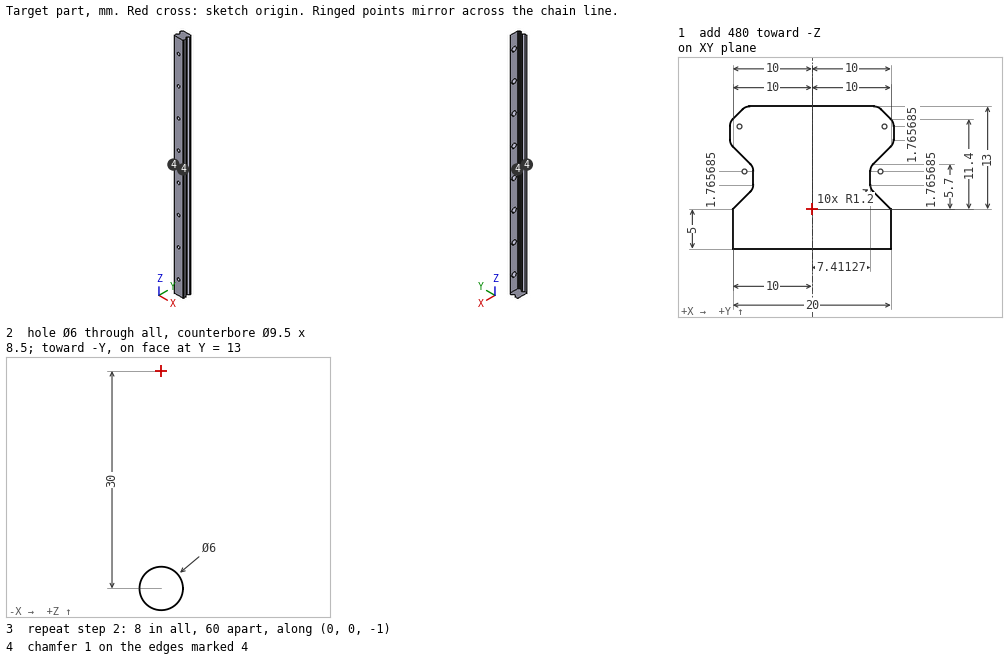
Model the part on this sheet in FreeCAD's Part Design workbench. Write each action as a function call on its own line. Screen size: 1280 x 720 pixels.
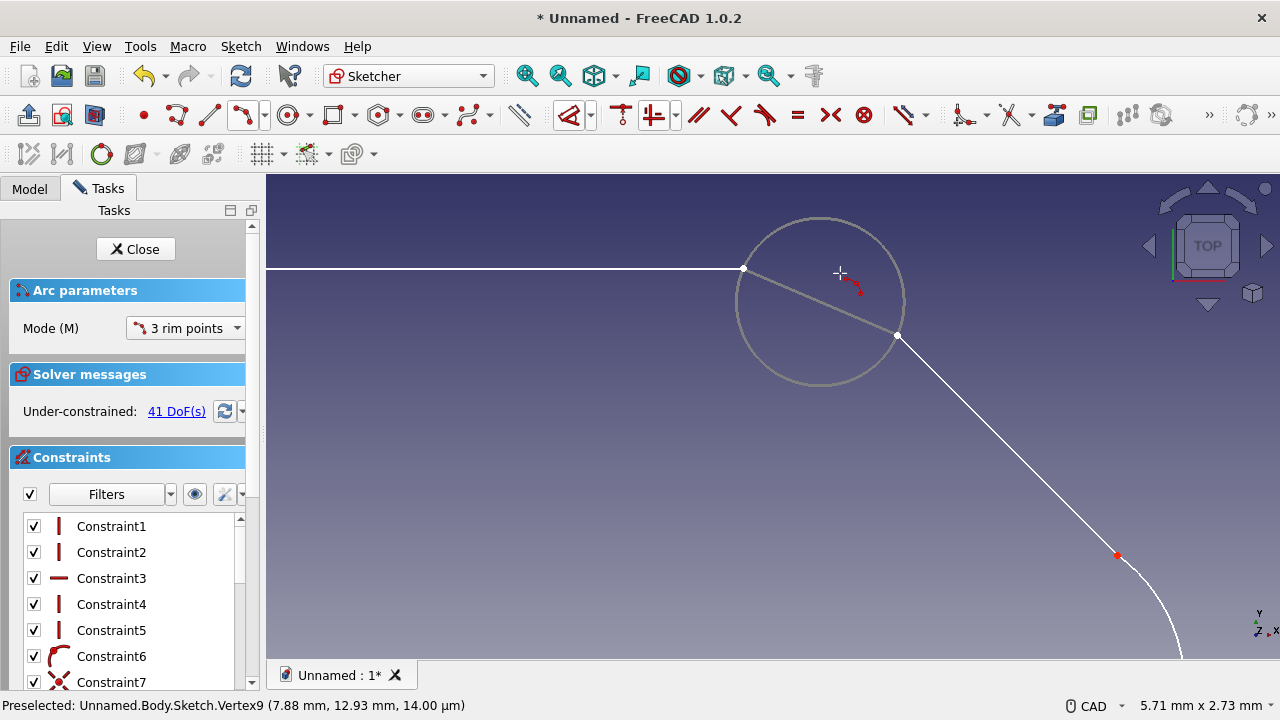
click(829, 274)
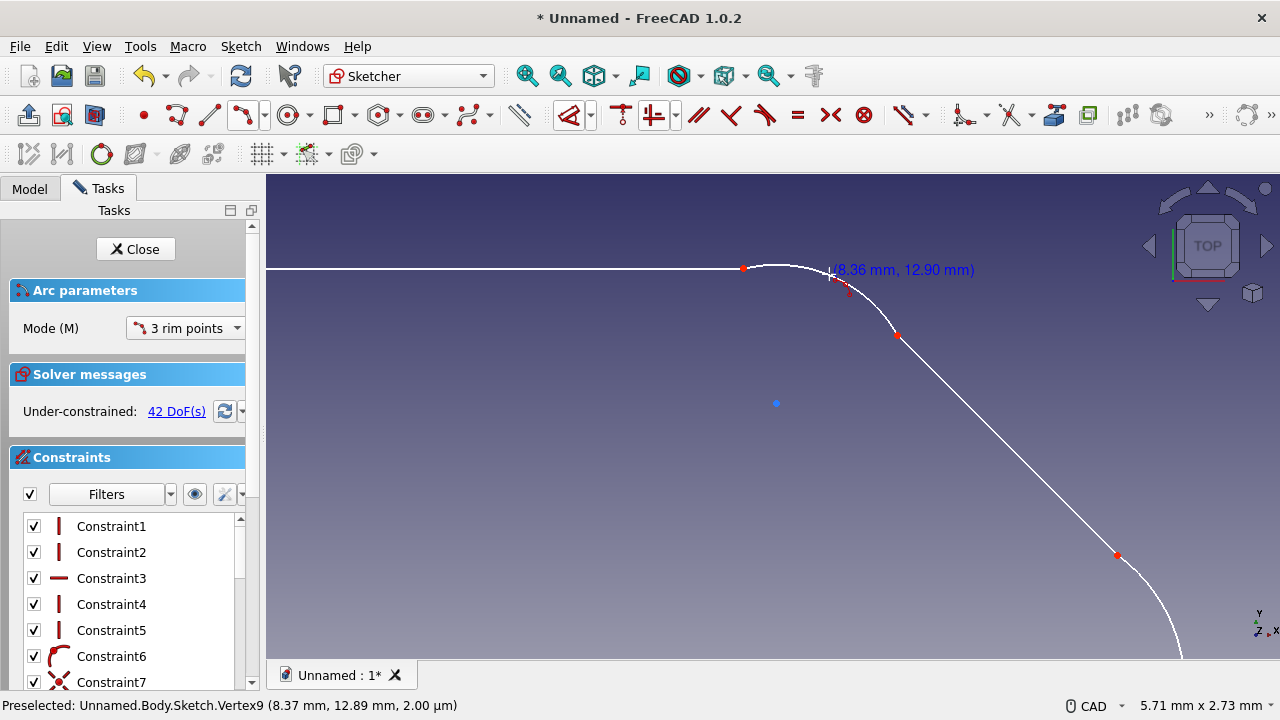
scroll(840, 273, down, 12)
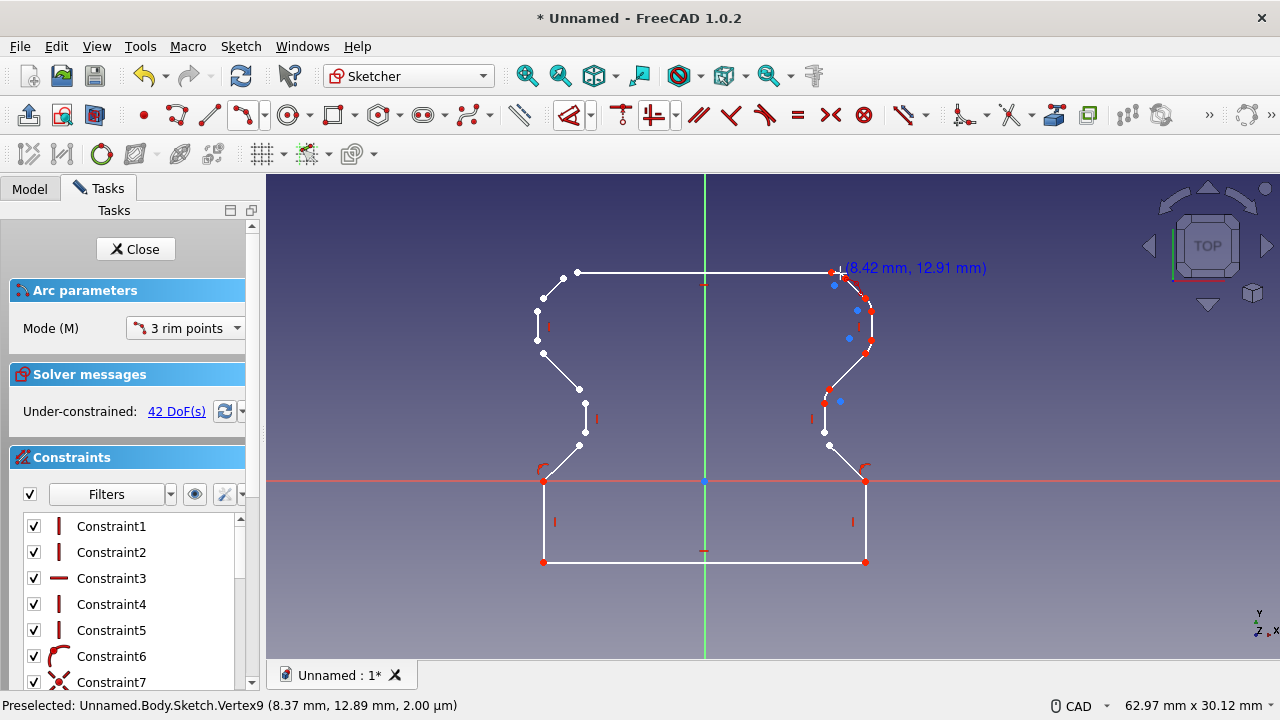
click(578, 273)
click(564, 279)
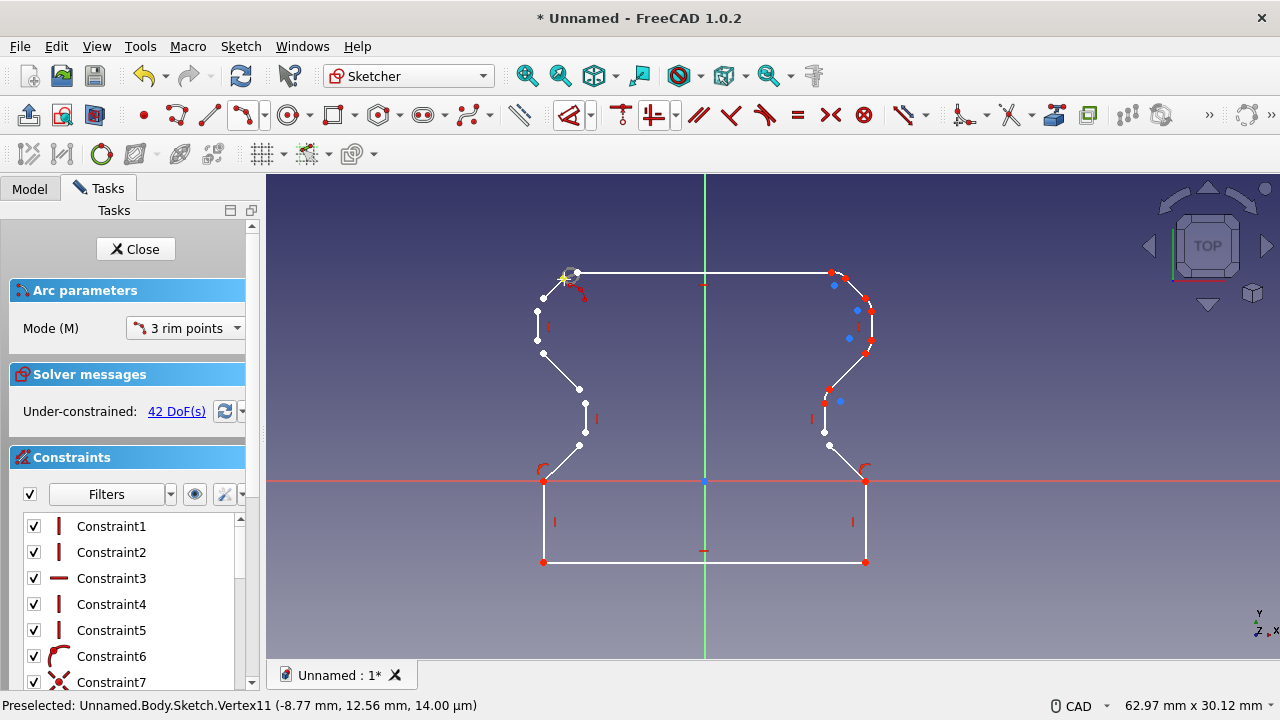
scroll(570, 273, up, 12)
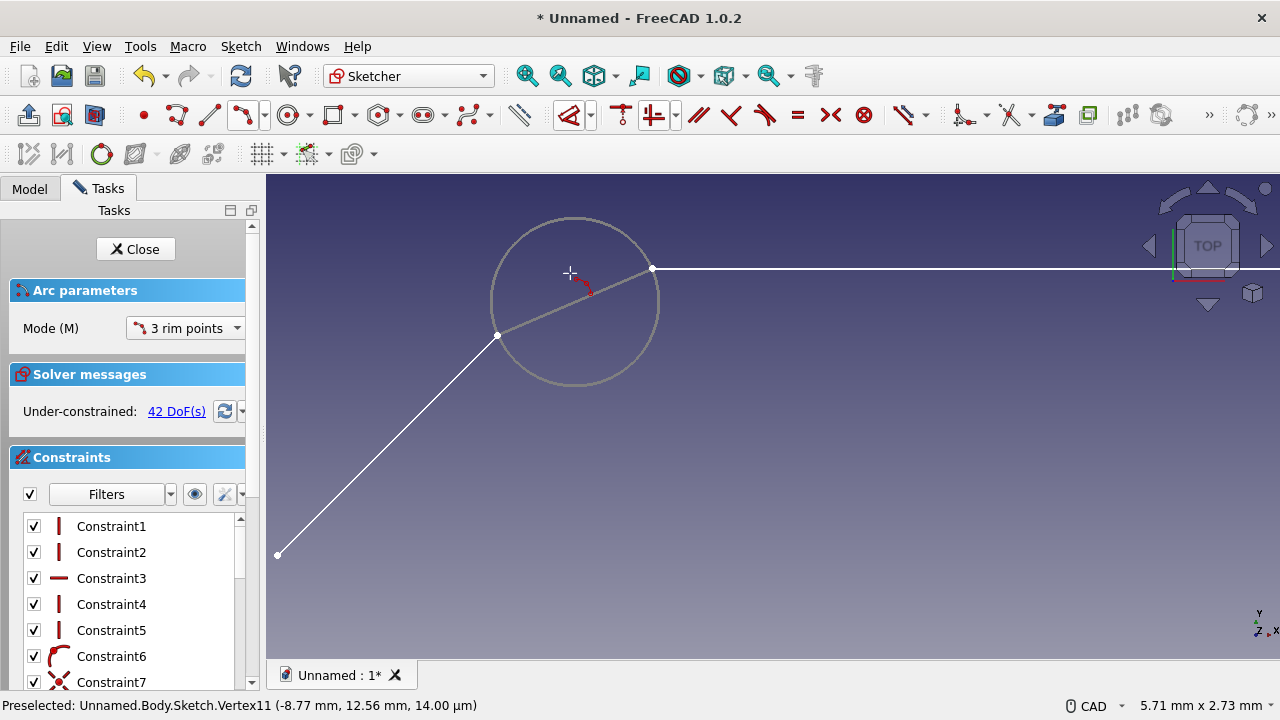
click(570, 274)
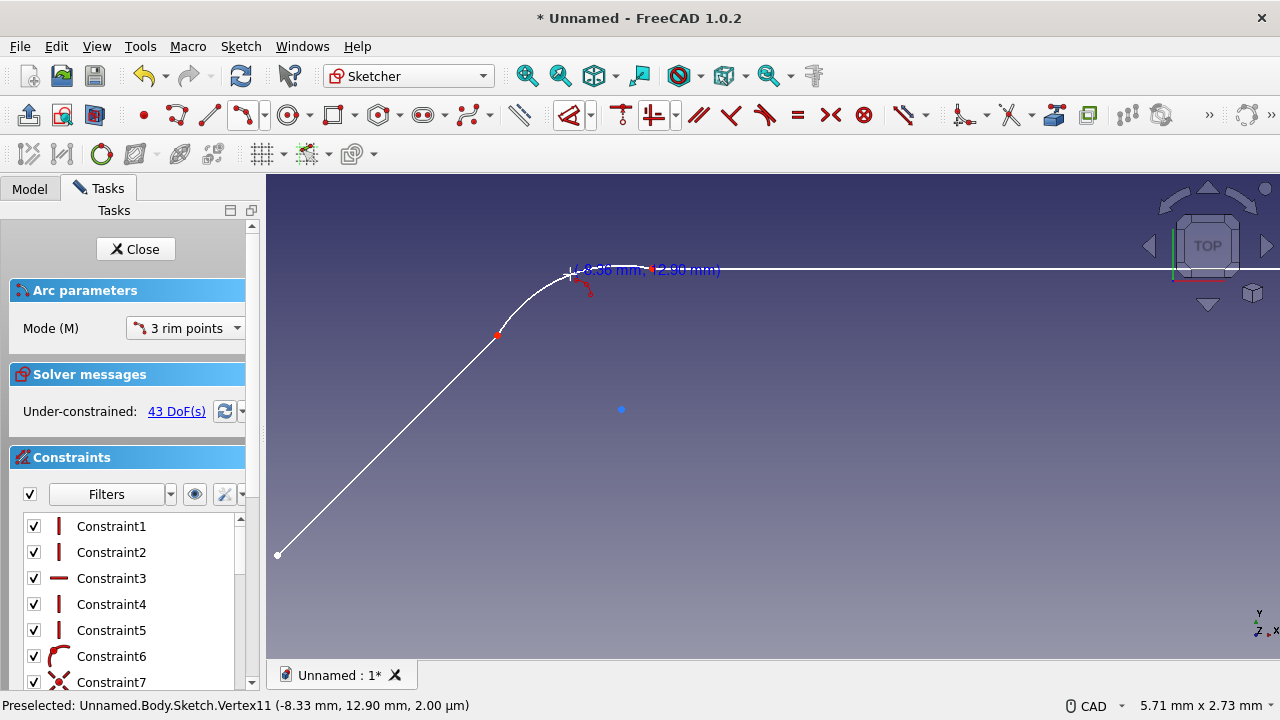
scroll(570, 273, down, 12)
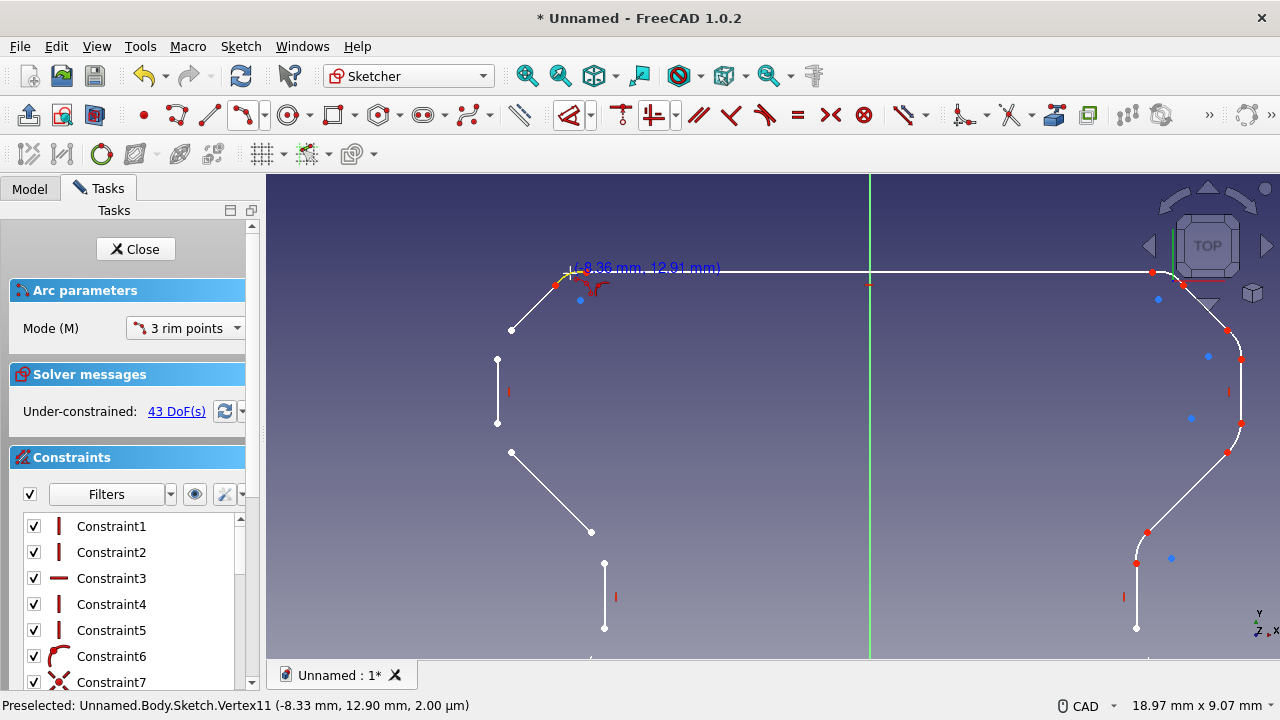
click(544, 299)
click(538, 312)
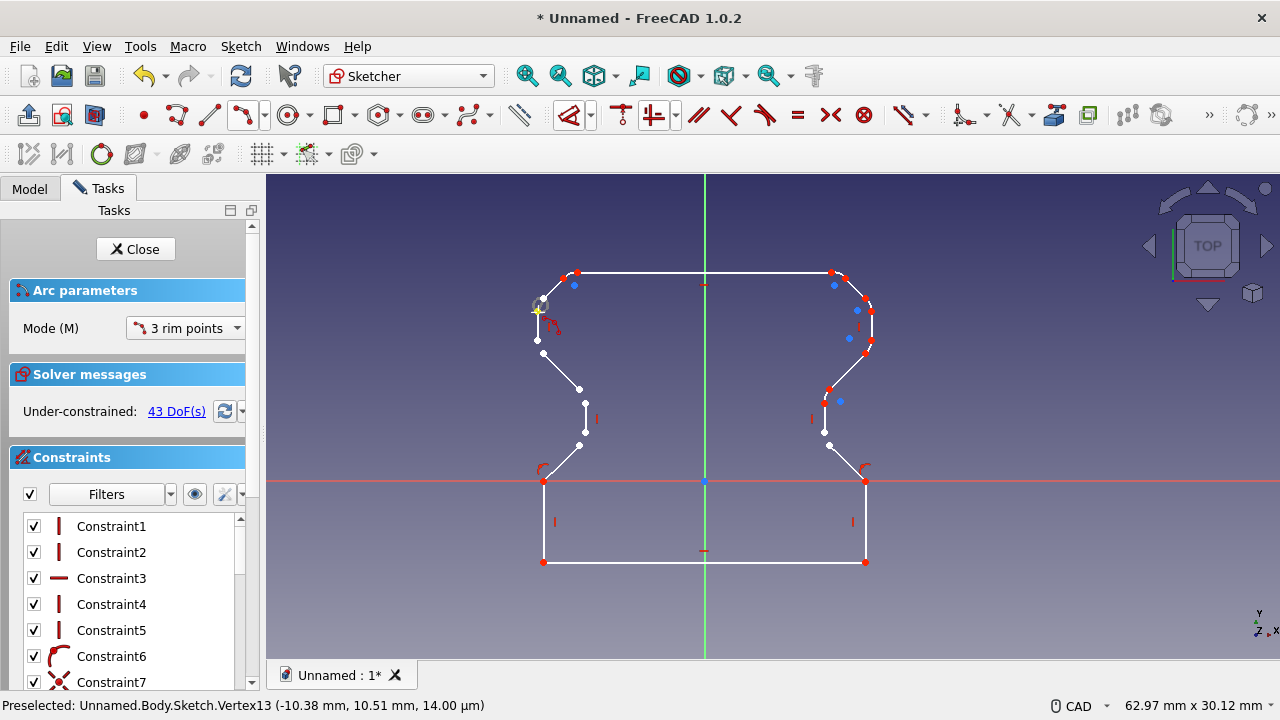
scroll(540, 304, up, 12)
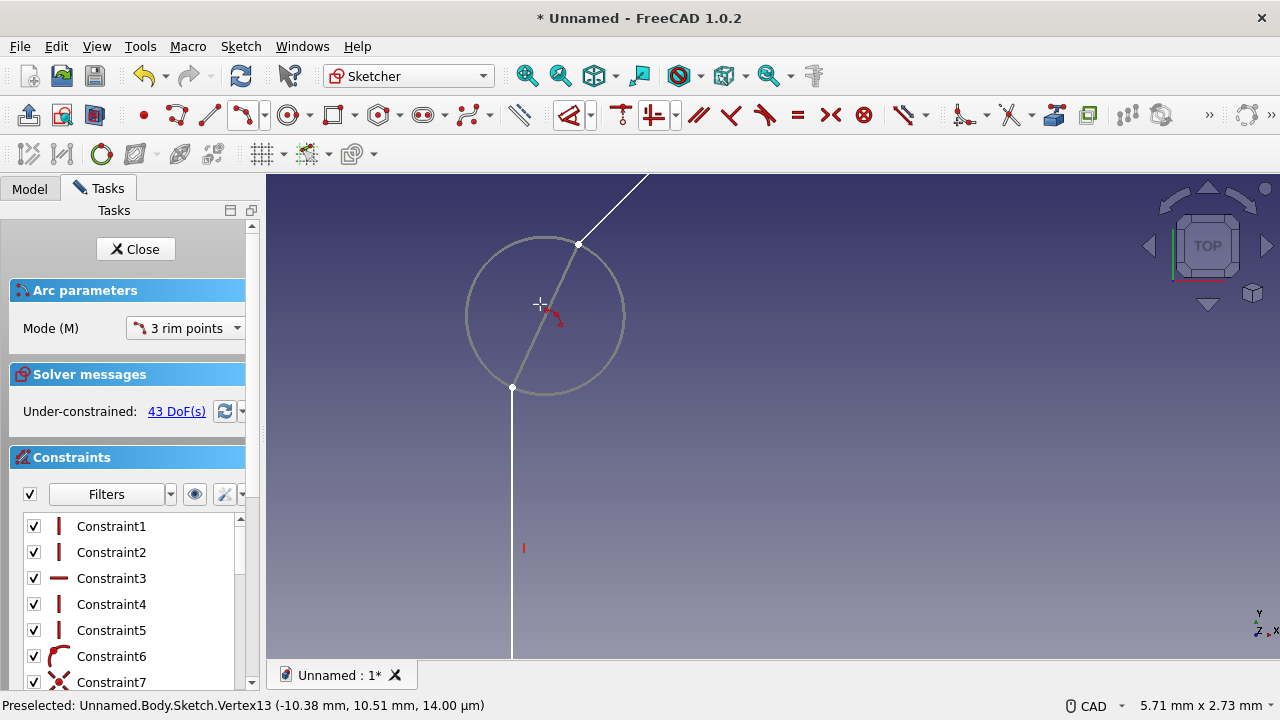
click(534, 299)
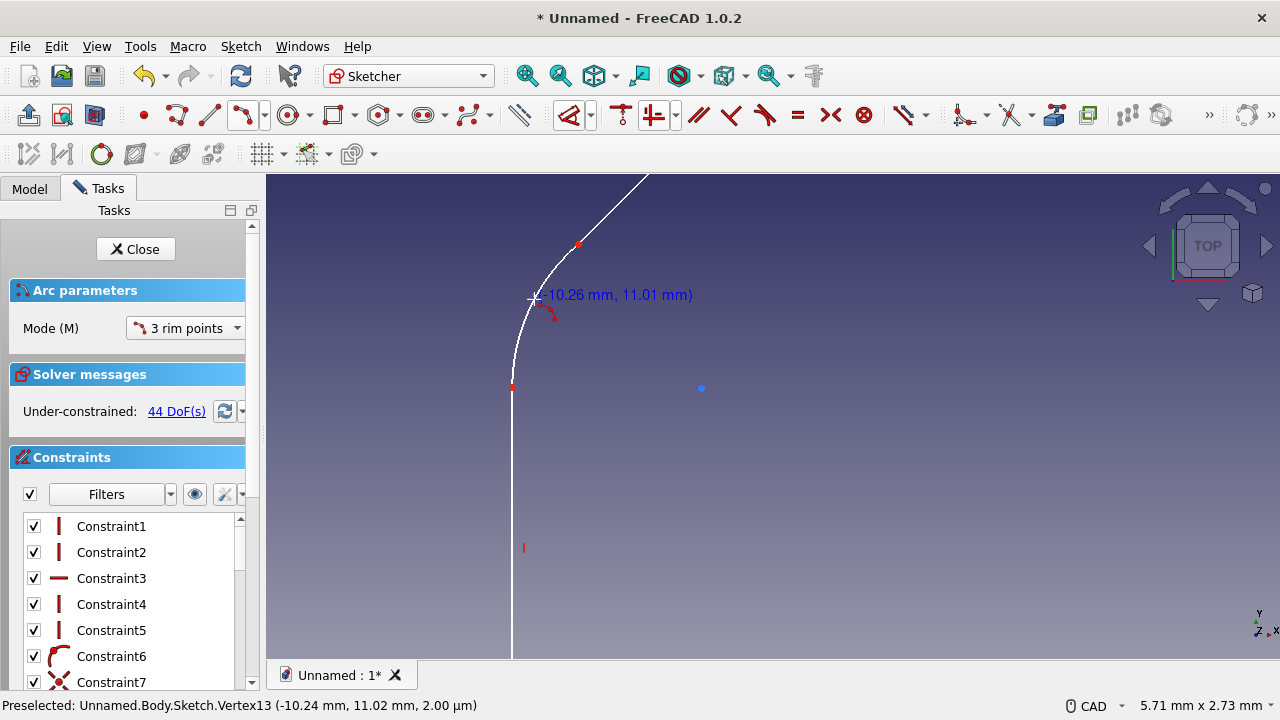
scroll(540, 304, down, 12)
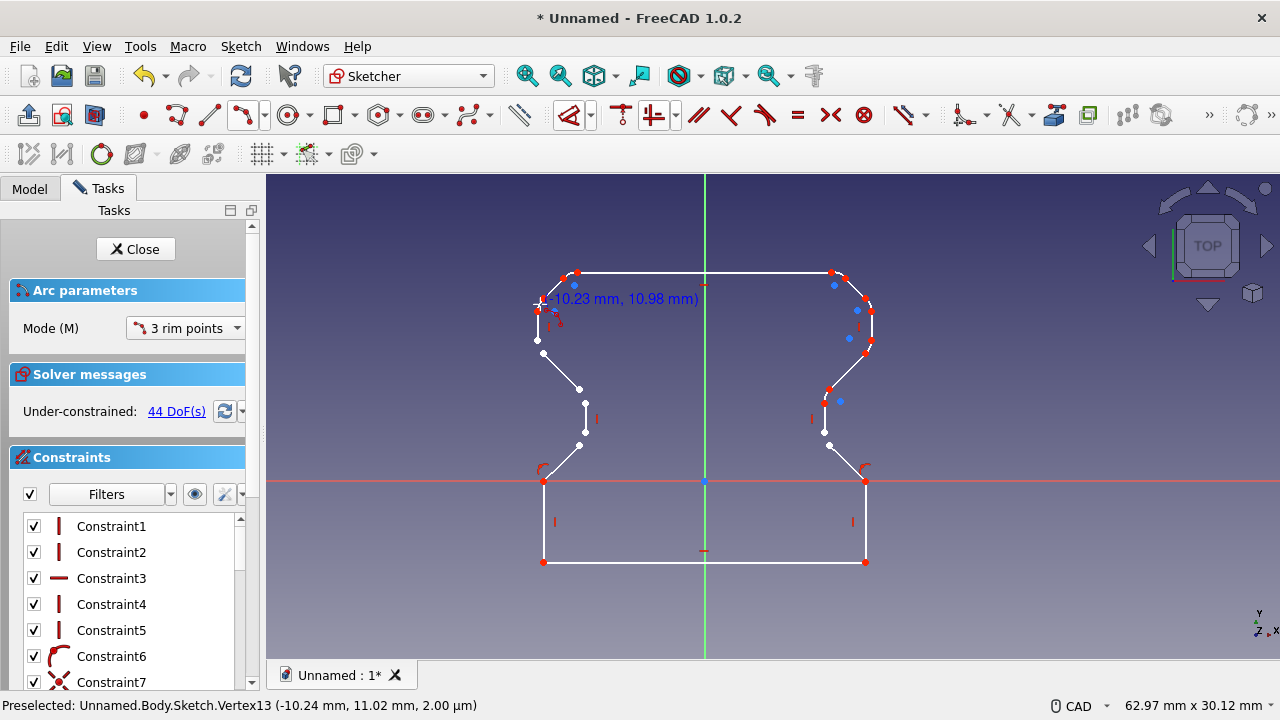
click(538, 341)
click(544, 354)